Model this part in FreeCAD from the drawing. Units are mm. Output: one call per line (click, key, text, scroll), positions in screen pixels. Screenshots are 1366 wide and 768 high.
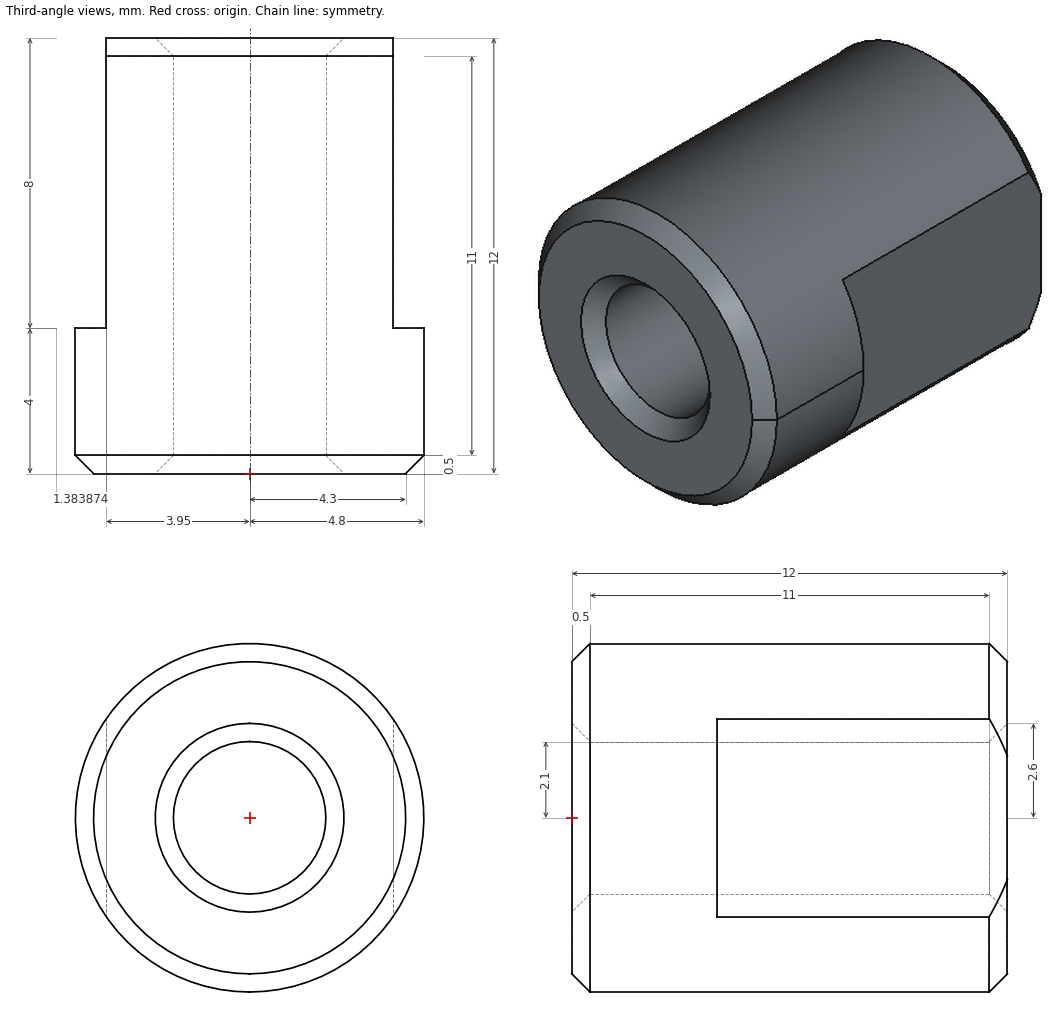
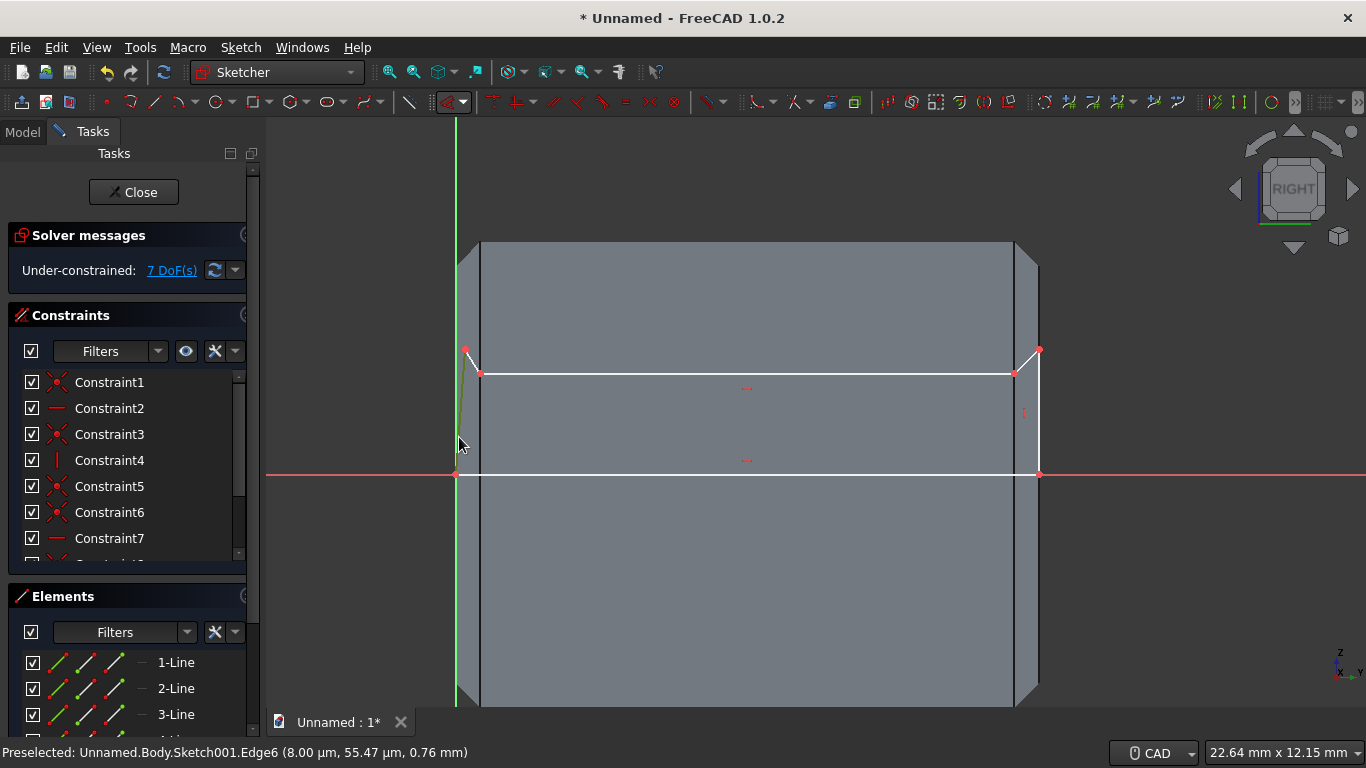
click(536, 102)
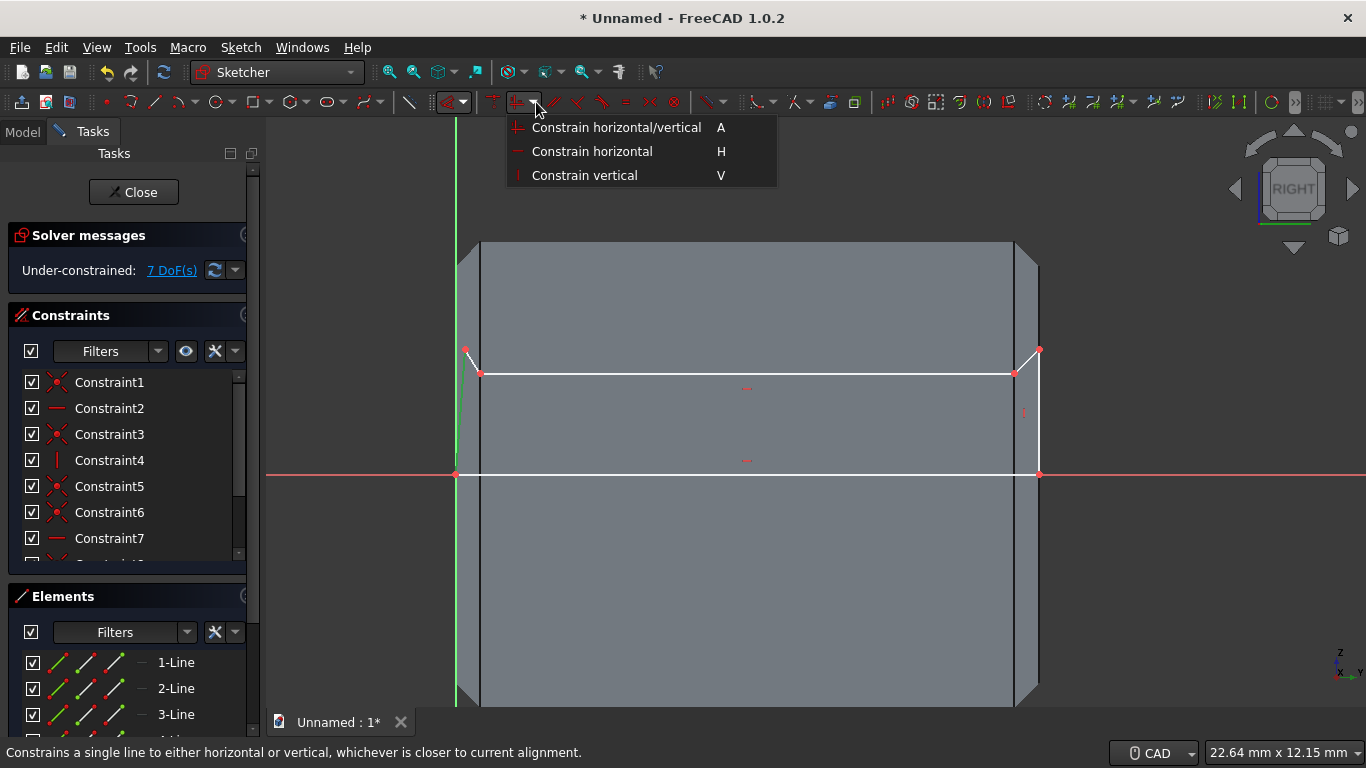
click(642, 175)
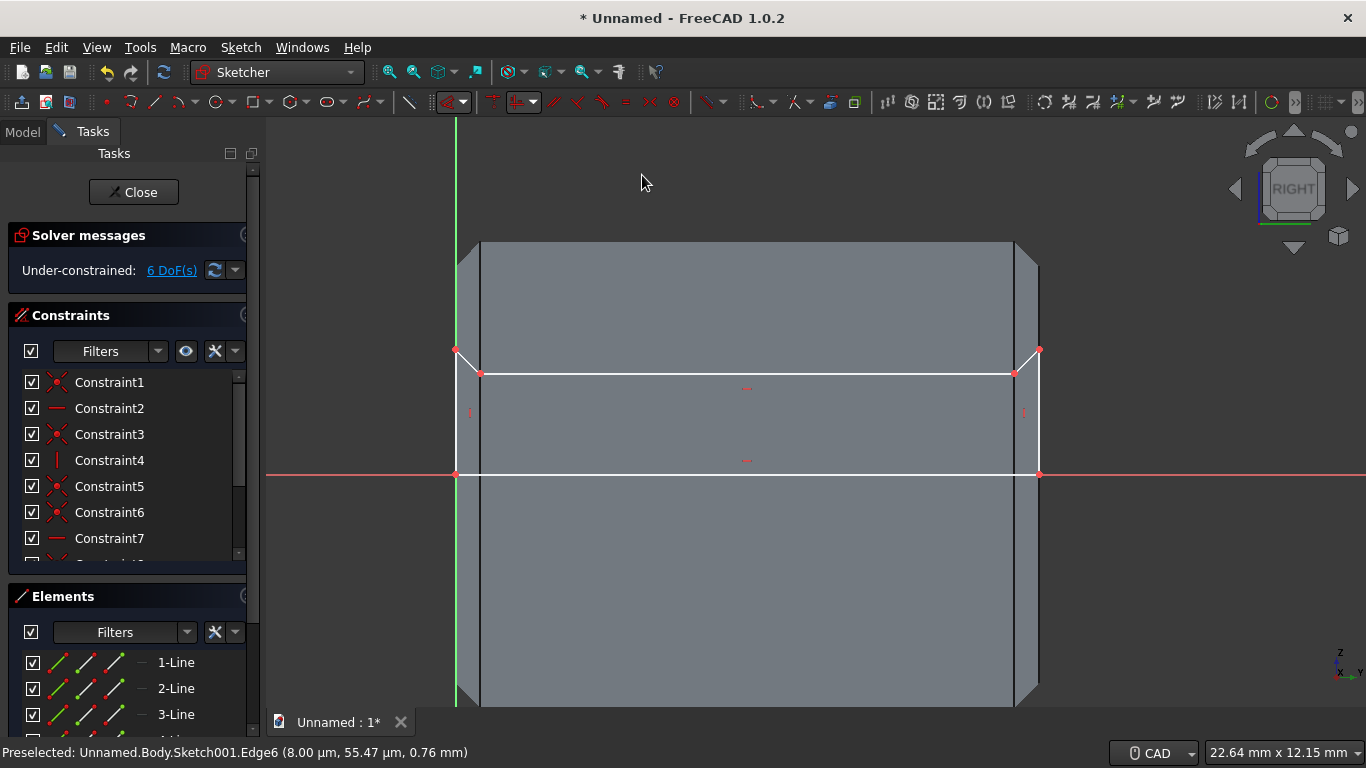
click(631, 475)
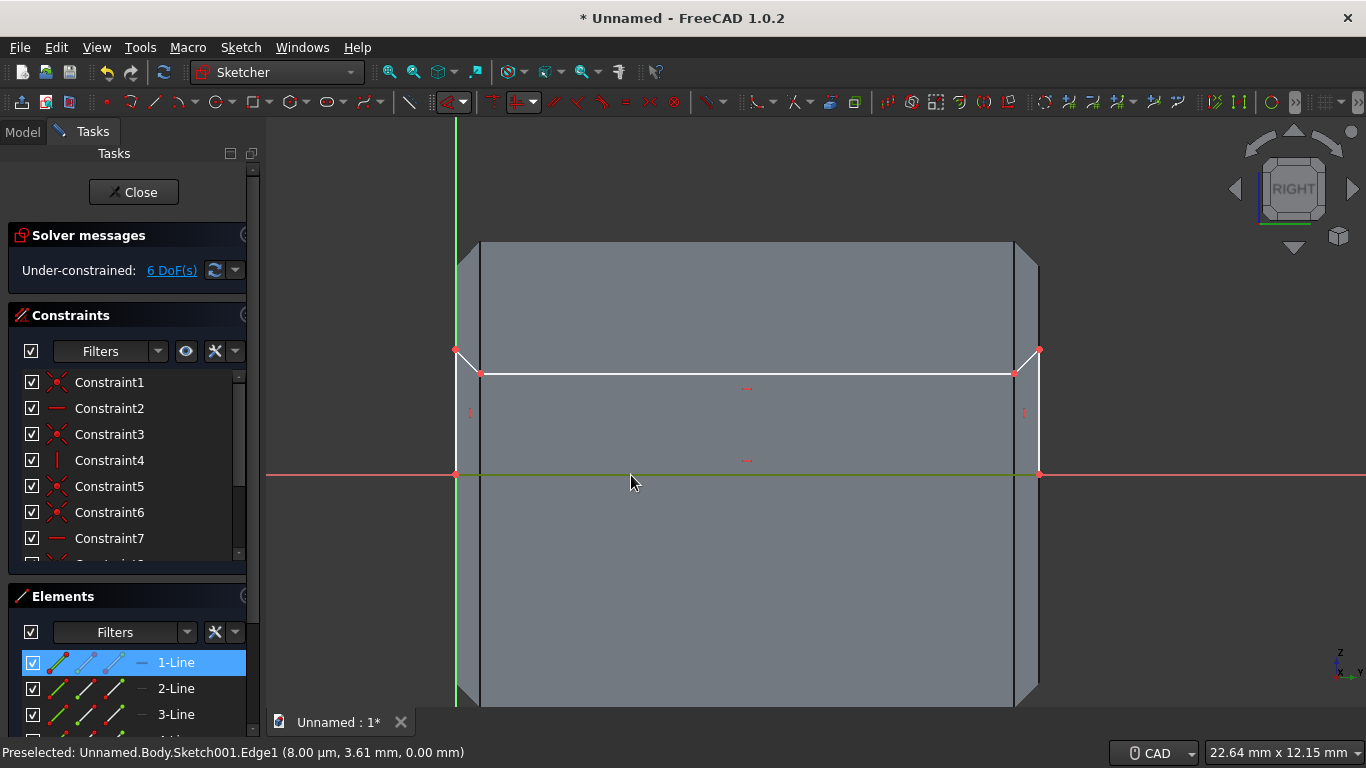
key(l)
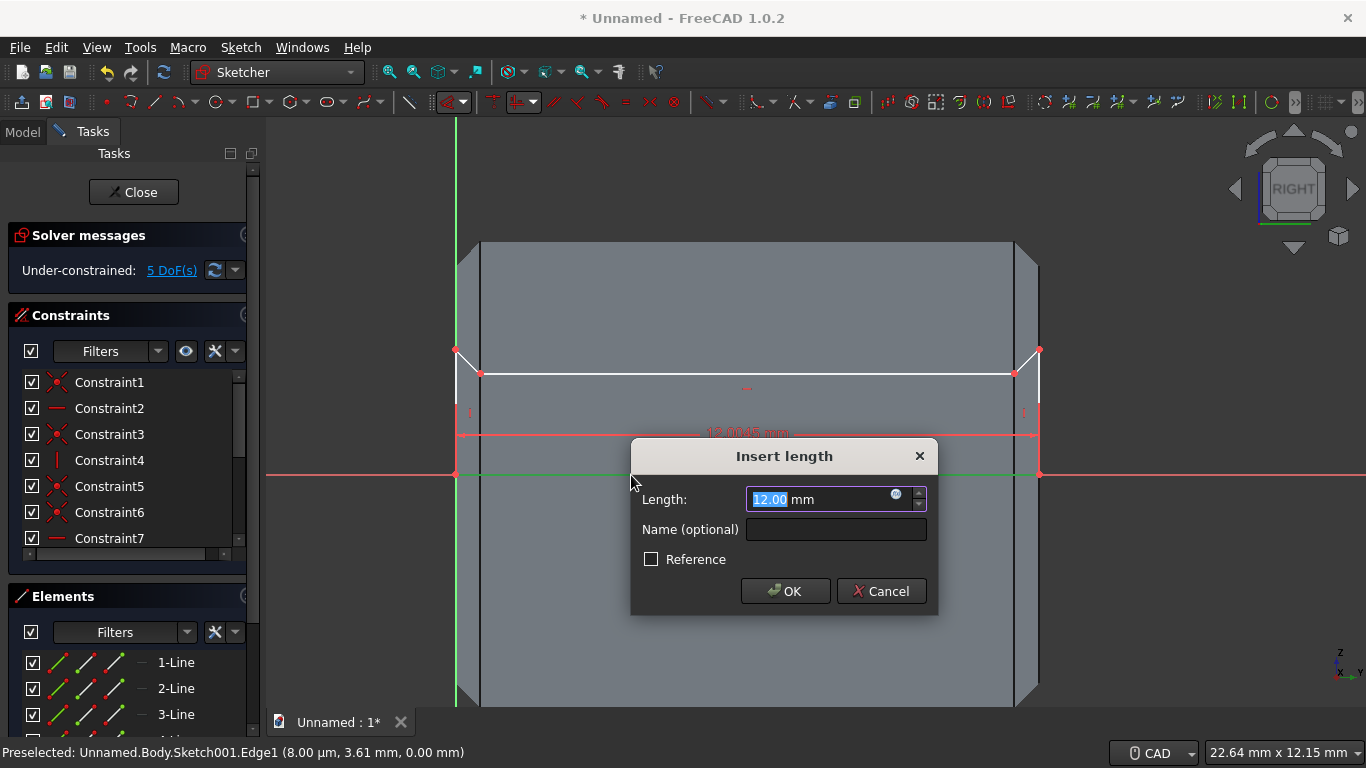
text(12)
key(Return)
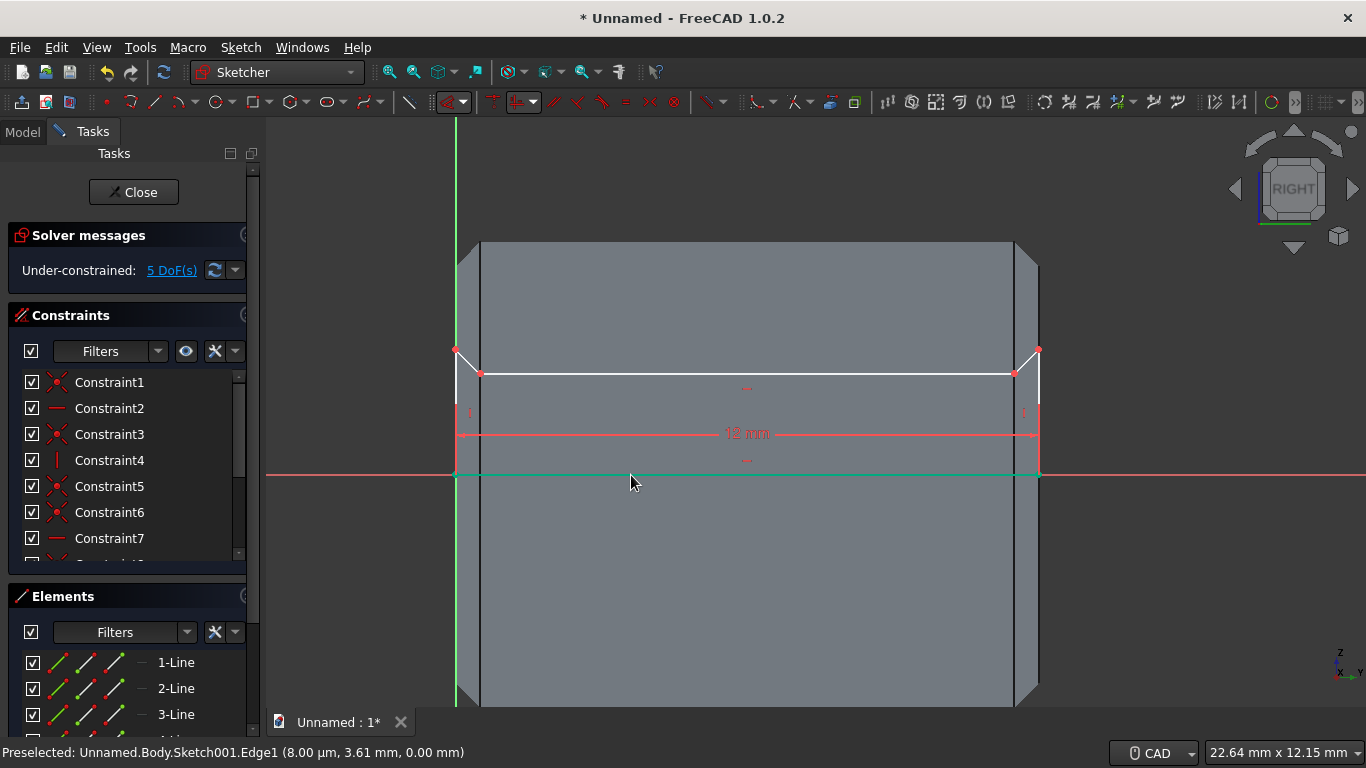
click(854, 374)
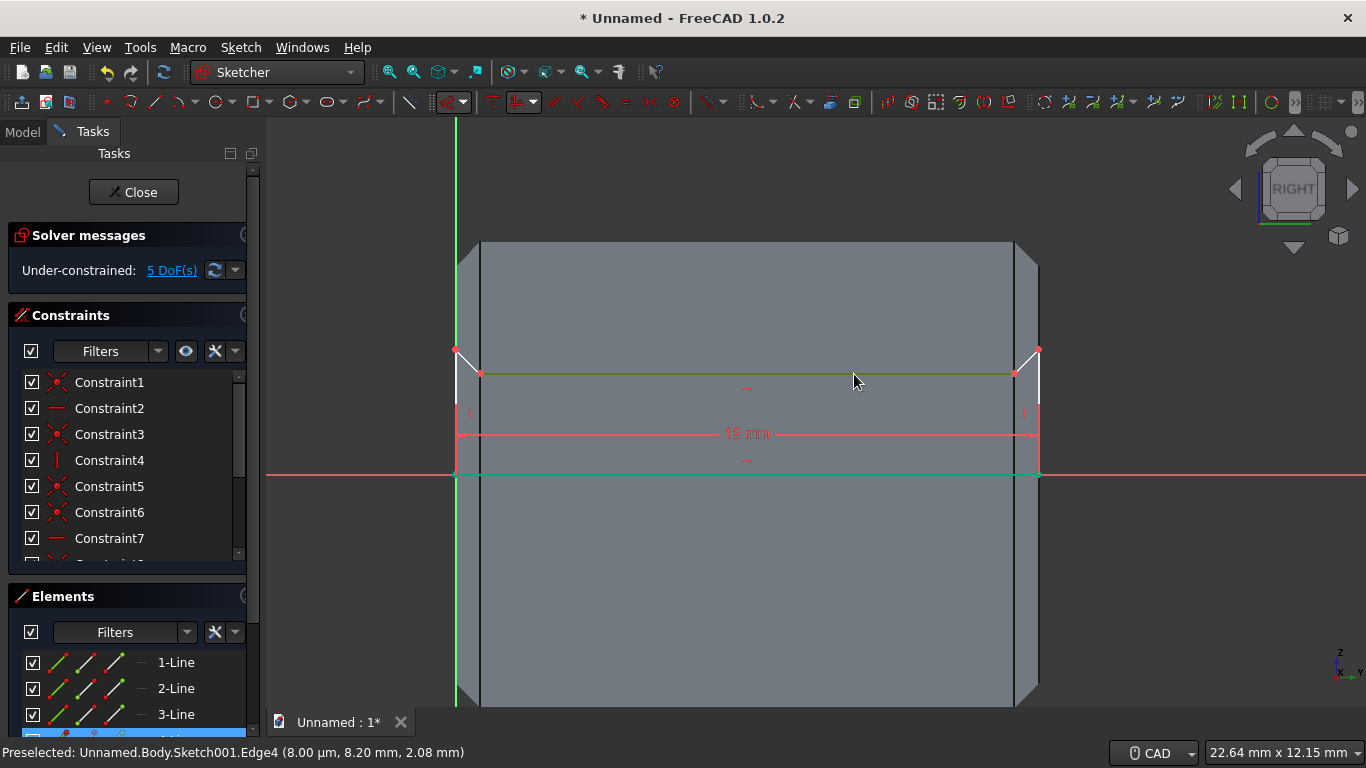
click(466, 102)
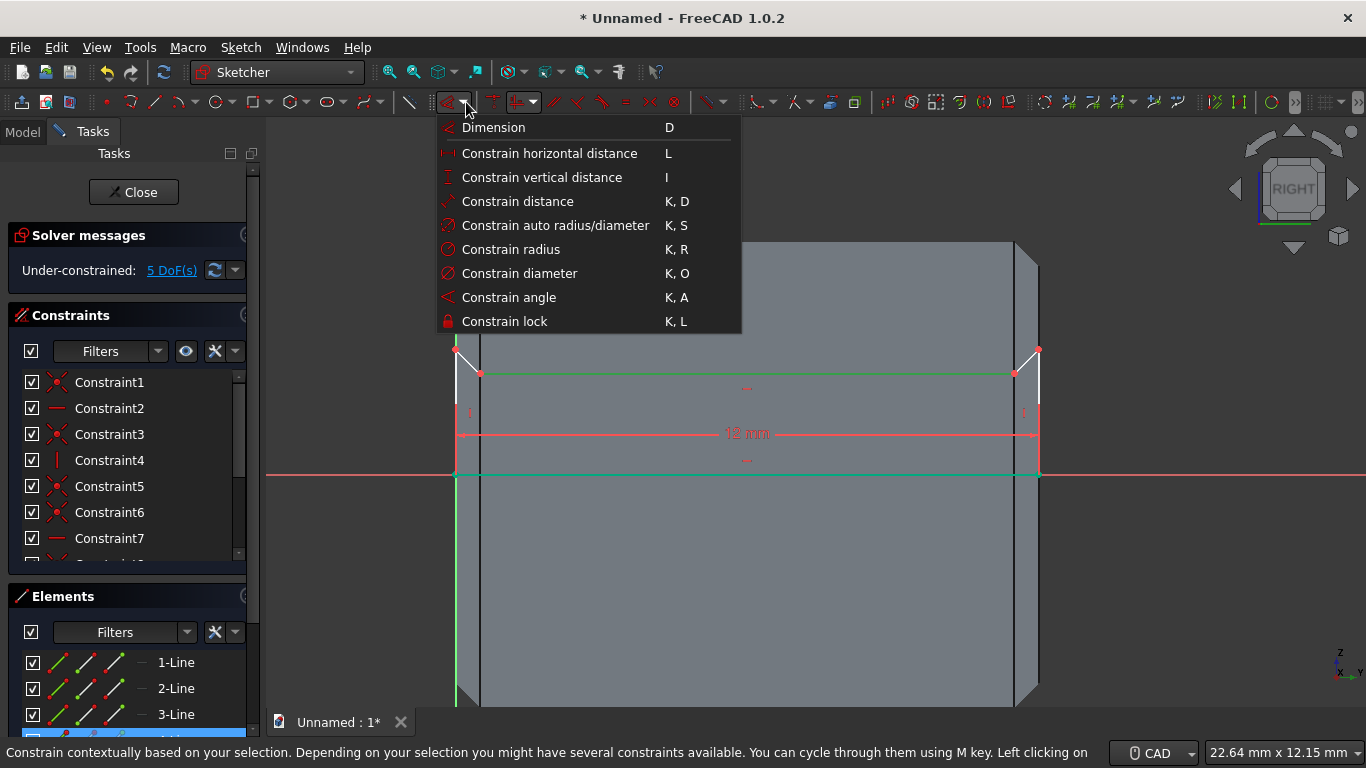
click(589, 153)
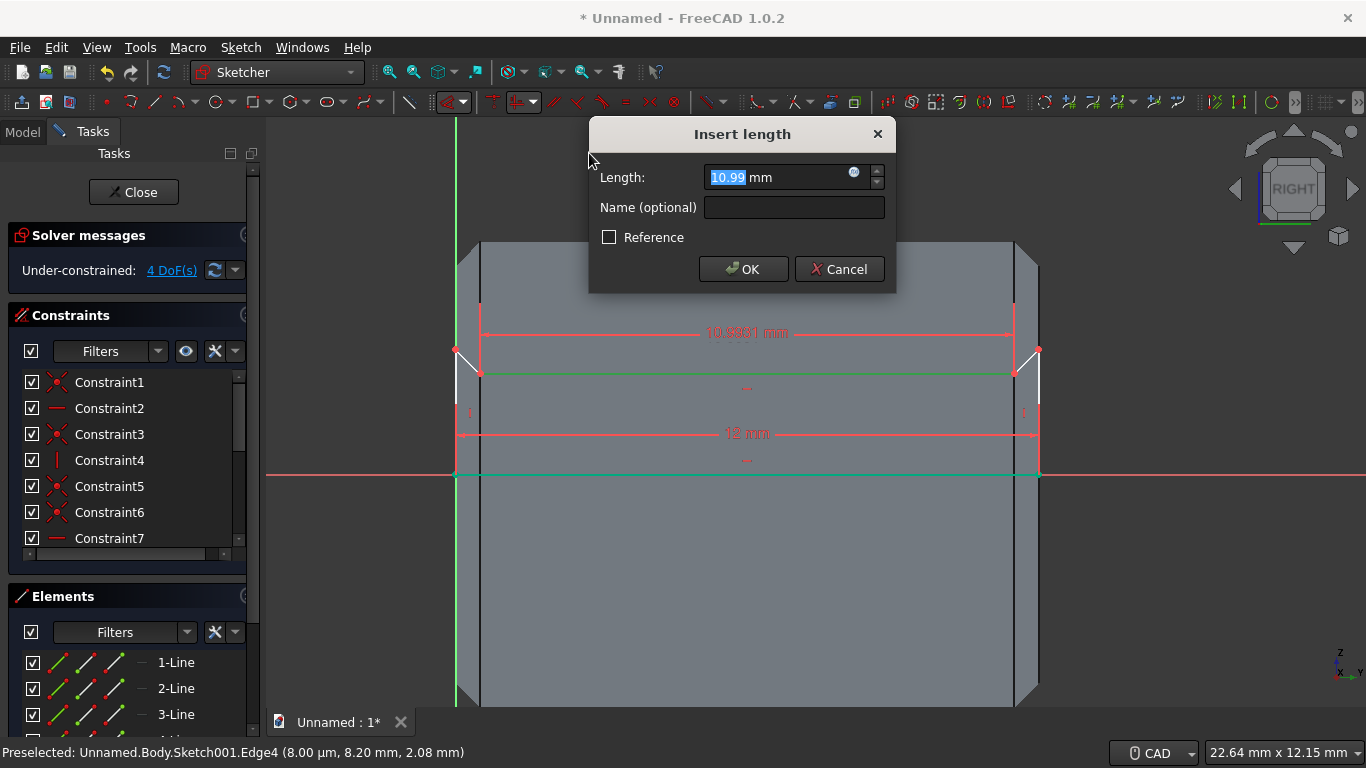
text(11)
key(Return)